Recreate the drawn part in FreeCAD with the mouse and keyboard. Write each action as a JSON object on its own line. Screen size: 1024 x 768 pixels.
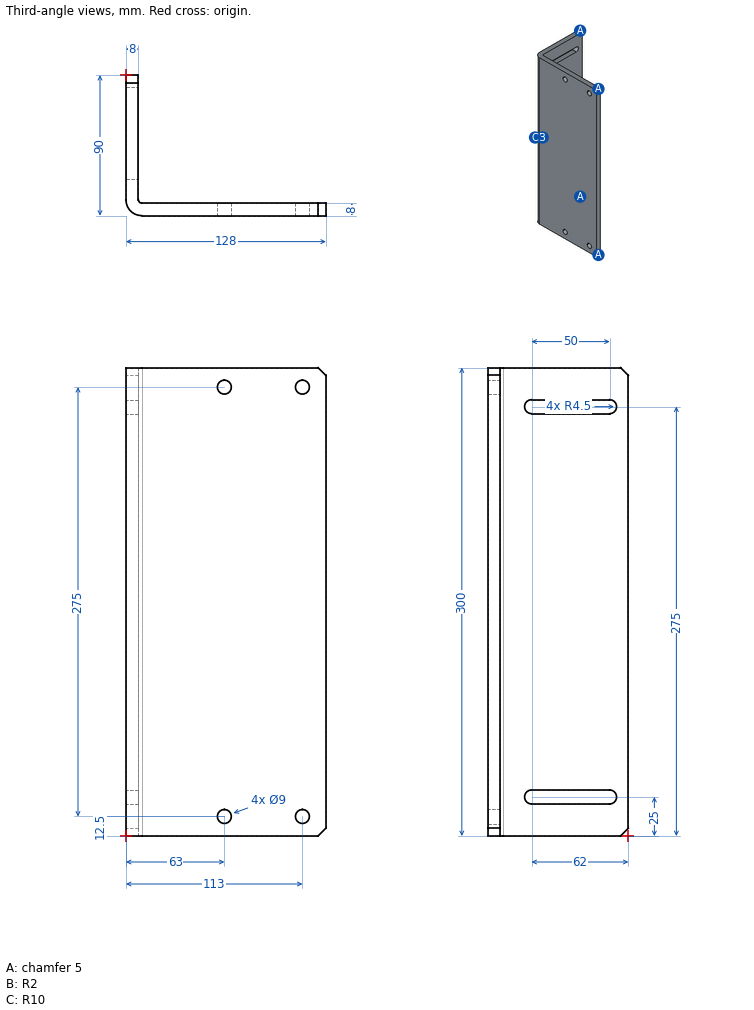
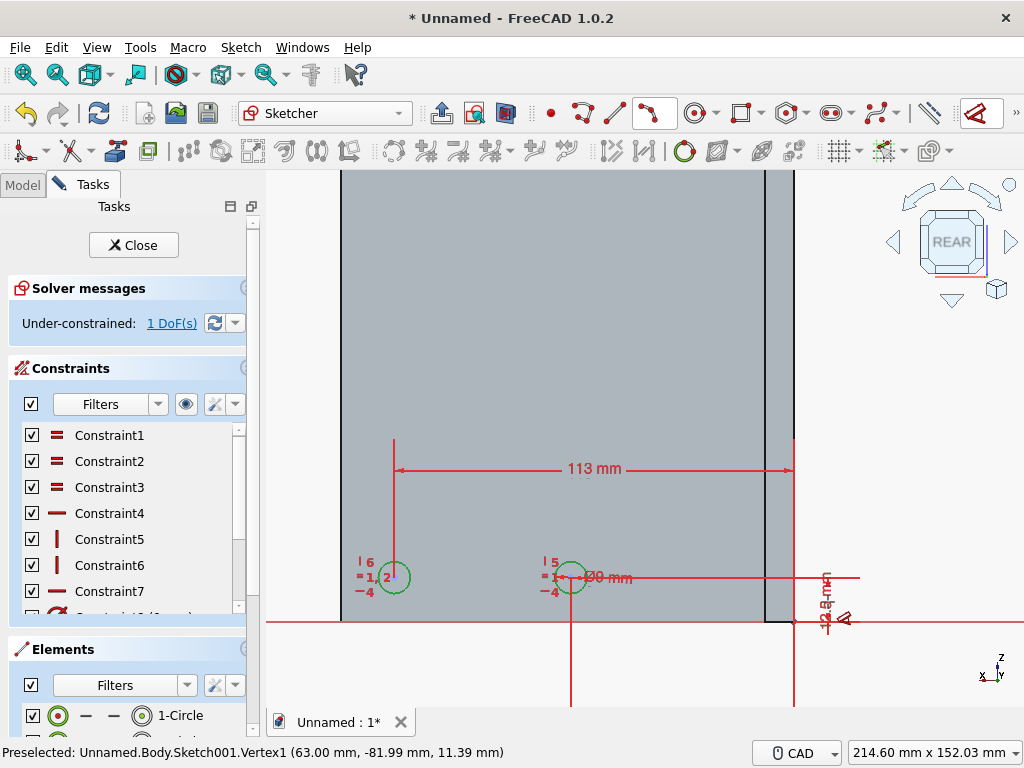
{"action": "left_click", "coordinate": [571, 578]}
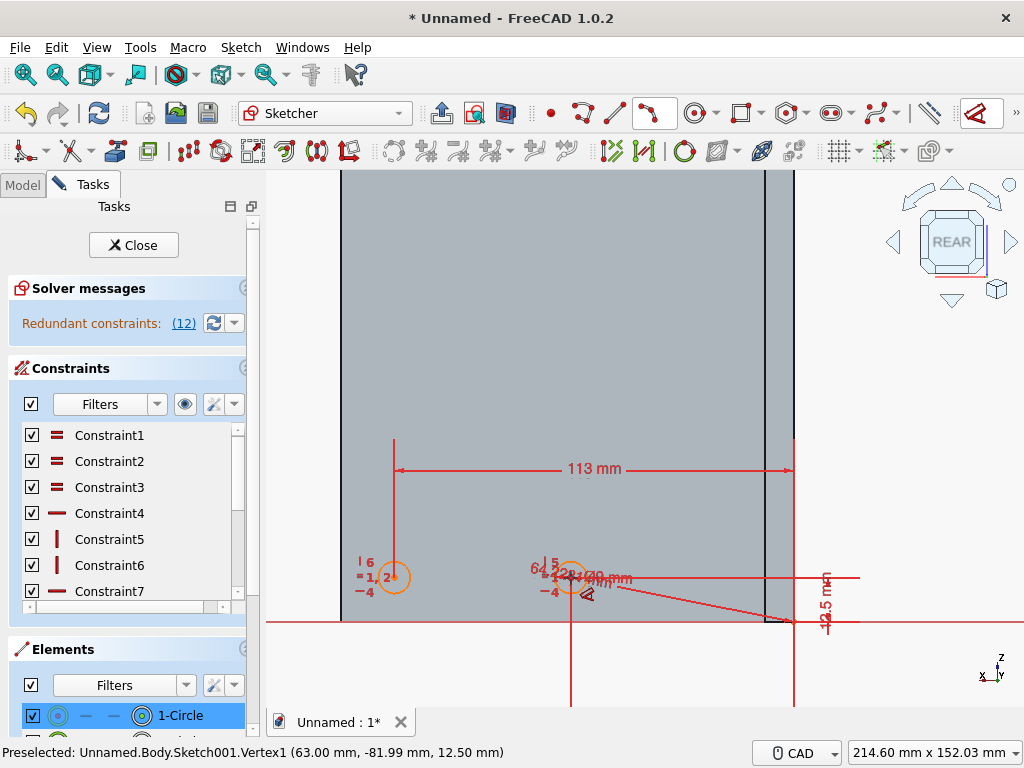
{"action": "scroll", "coordinate": [572, 582], "scroll_direction": "down", "scroll_amount": 6}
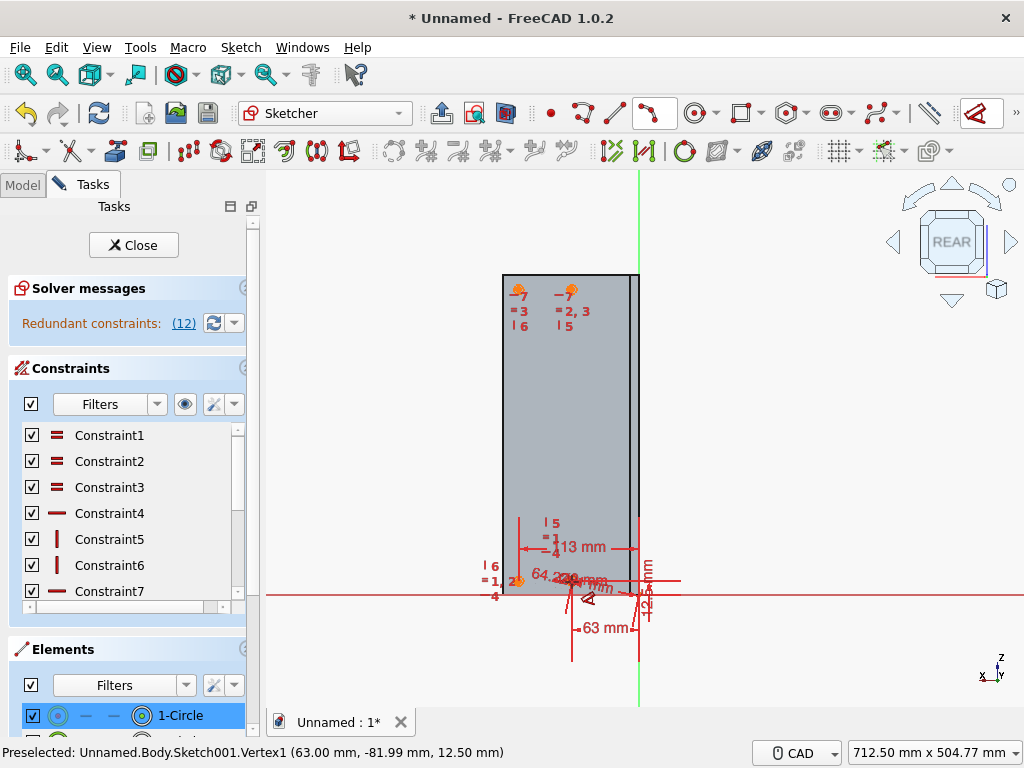
{"action": "left_click", "coordinate": [572, 290]}
{"action": "left_click", "coordinate": [538, 435]}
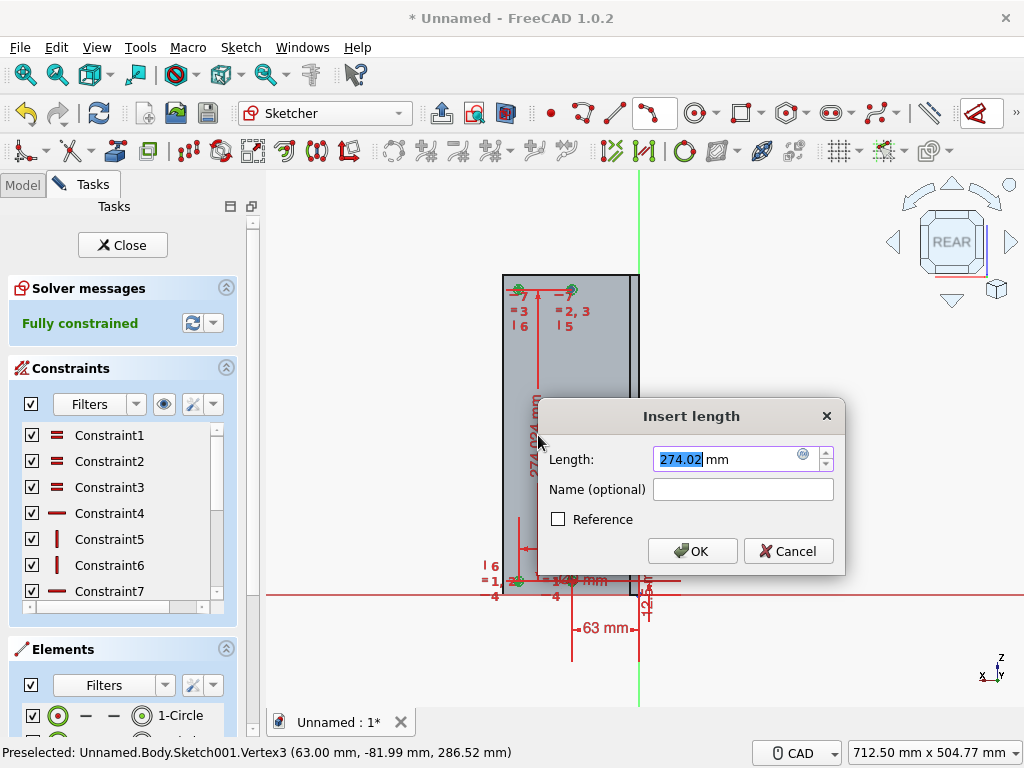
{"action": "type", "text": "275"}
{"action": "key", "text": "Return"}
{"action": "key", "text": "Escape"}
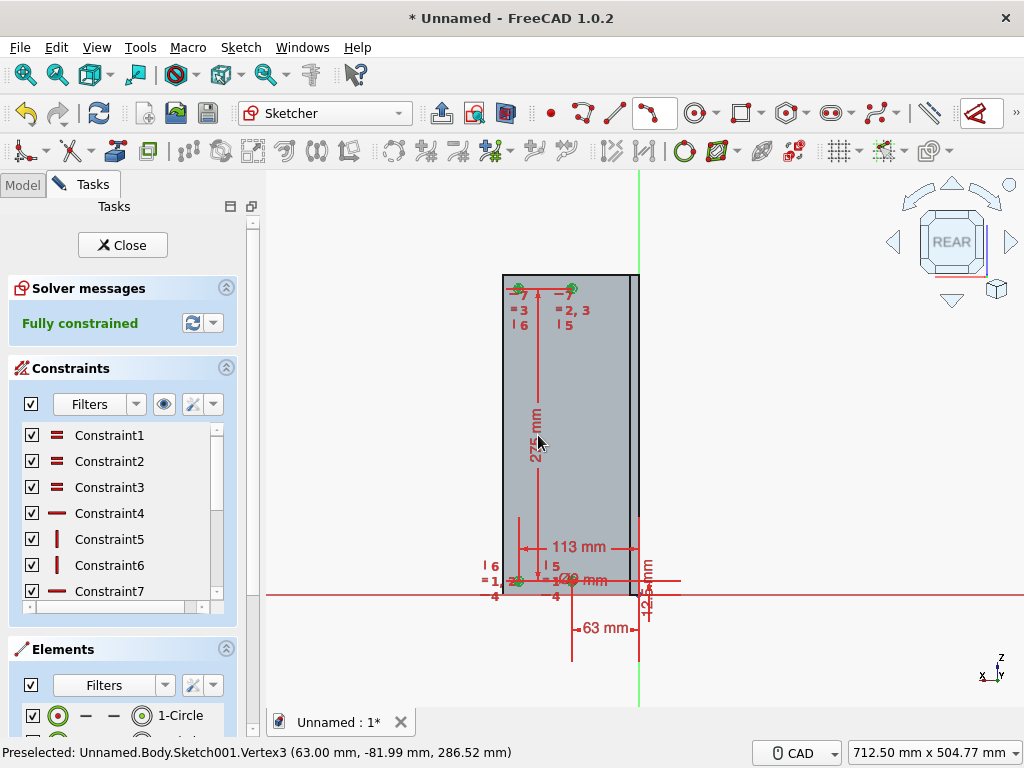
{"action": "left_click", "coordinate": [123, 245]}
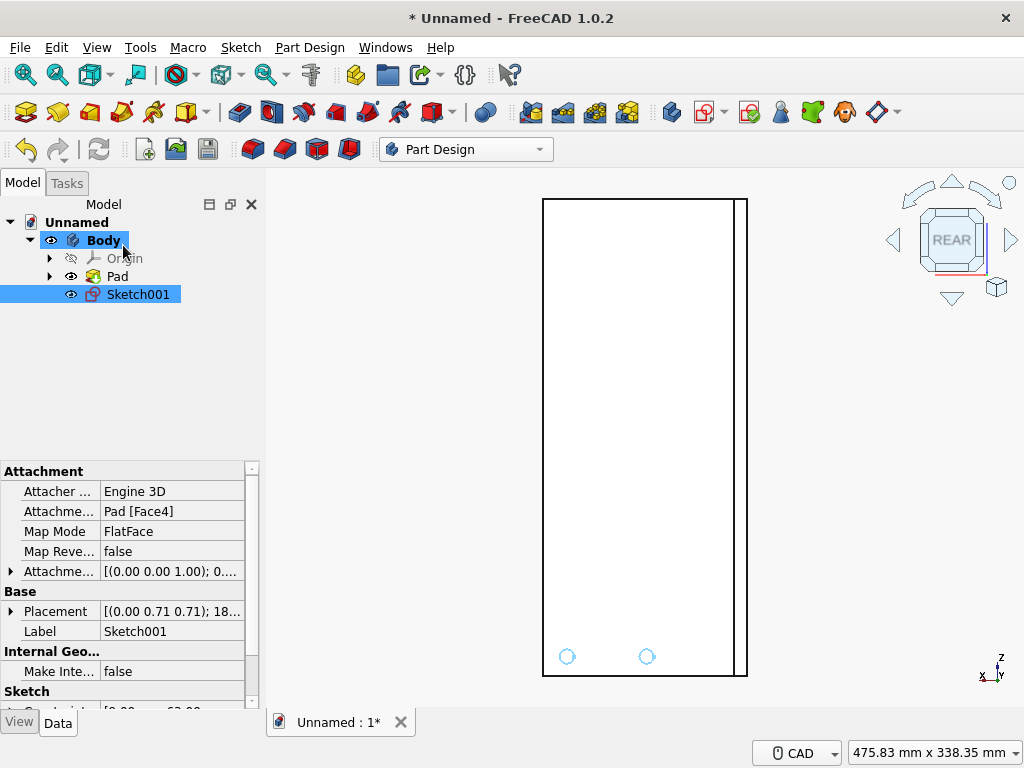
{"action": "left_click", "coordinate": [240, 112]}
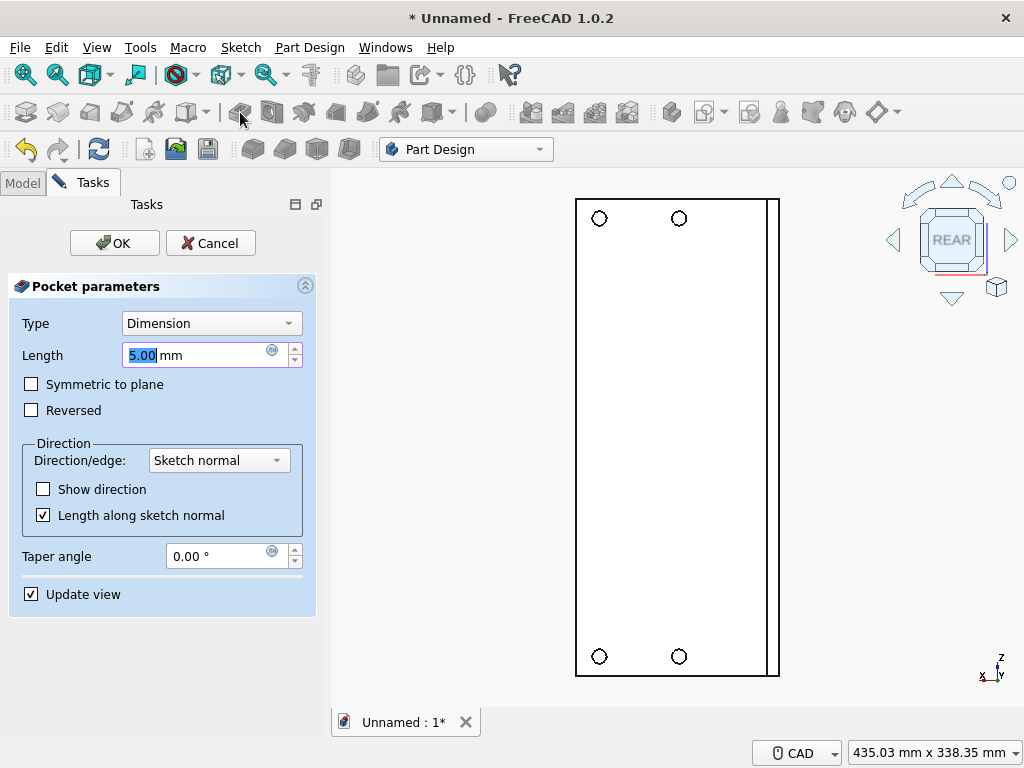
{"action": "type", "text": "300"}
{"action": "key", "text": "Tab"}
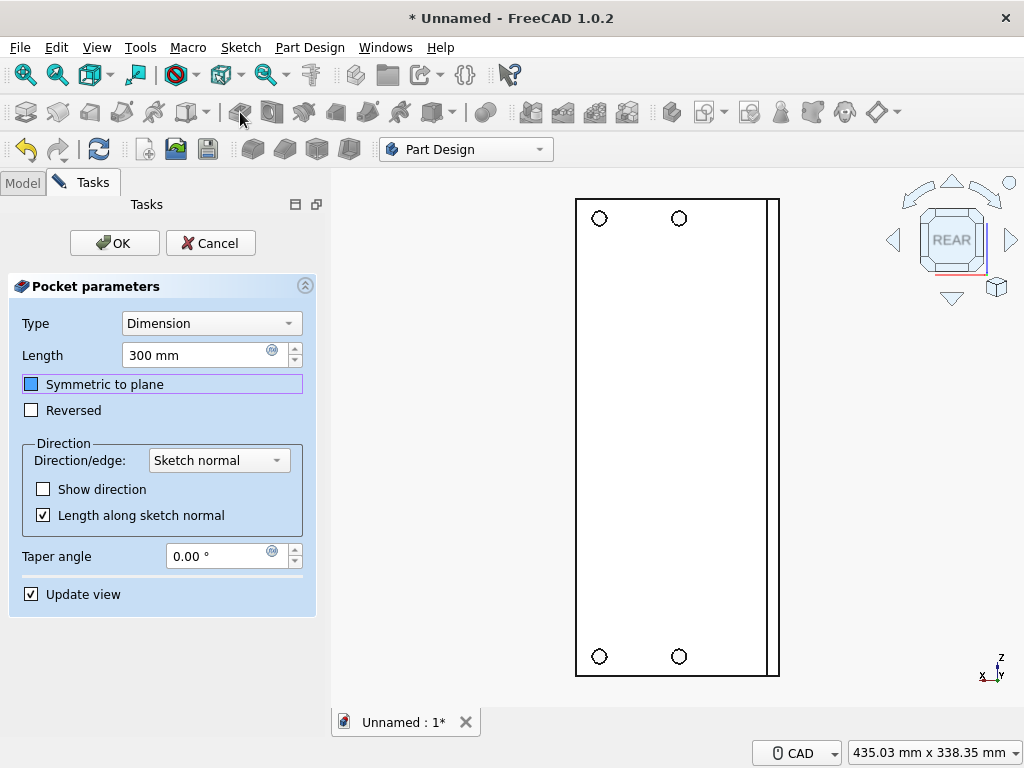
{"action": "left_click", "coordinate": [115, 243]}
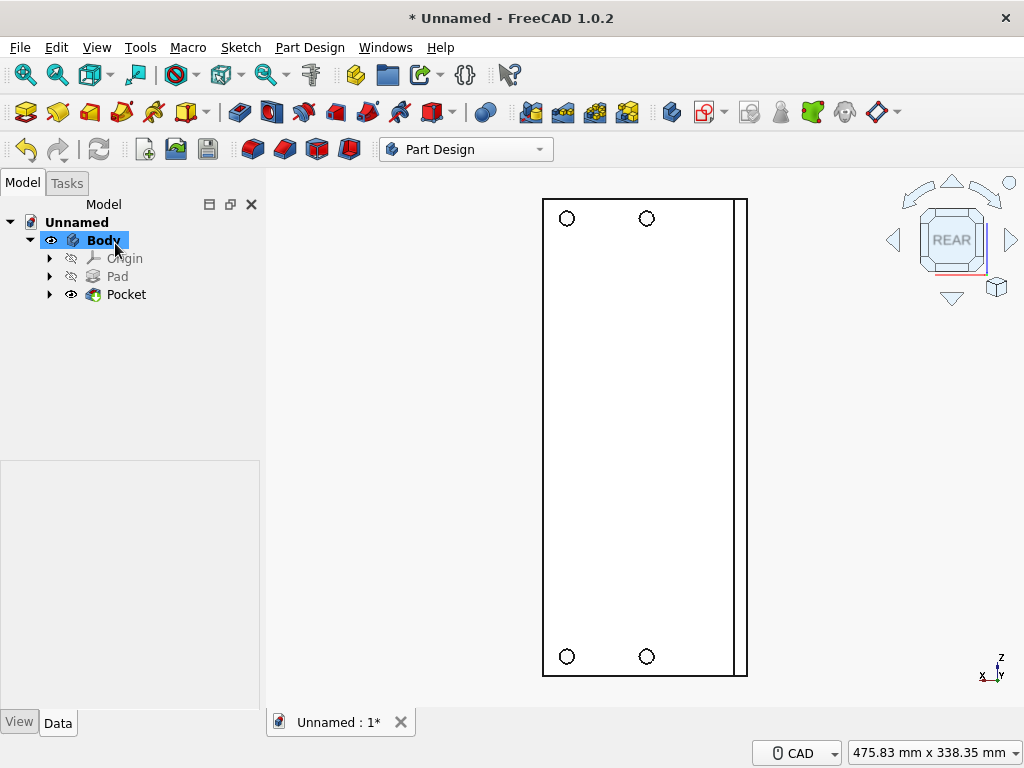
{"action": "key", "text": "0"}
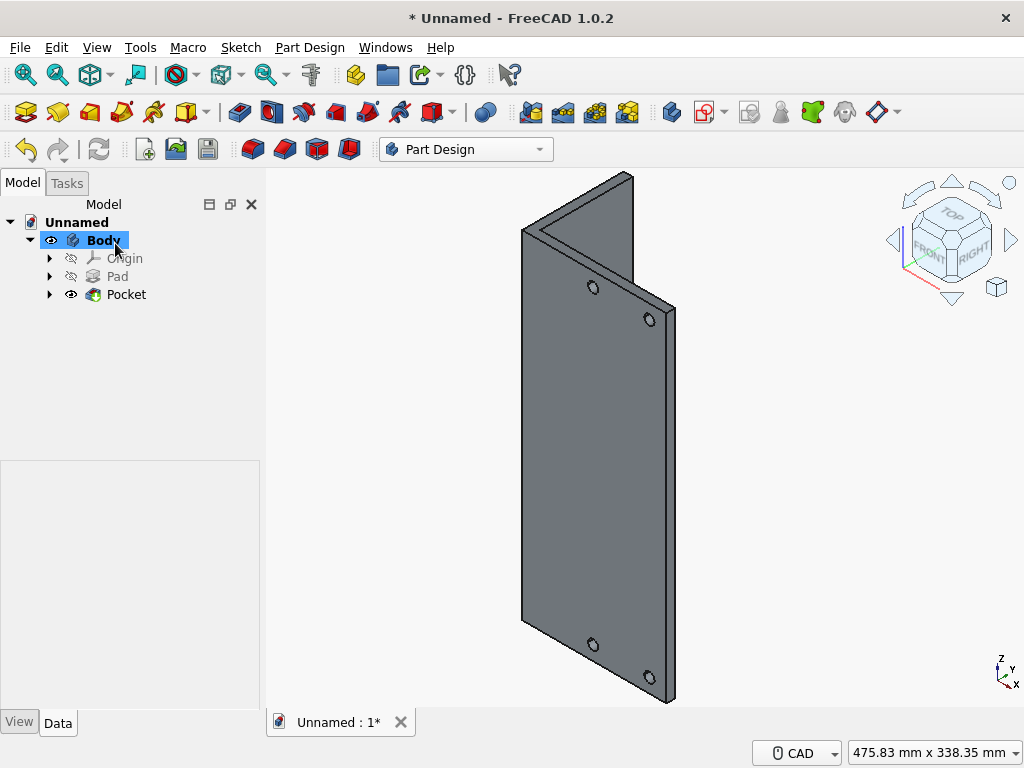
{"action": "key", "text": "3"}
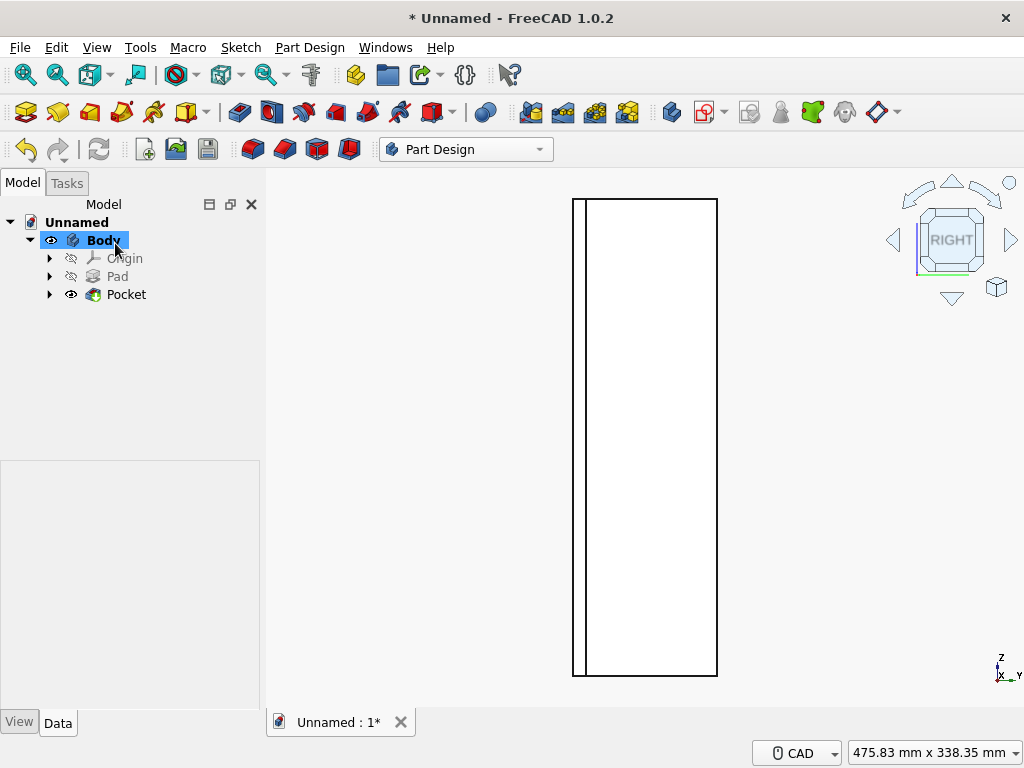
{"action": "left_click", "coordinate": [651, 300]}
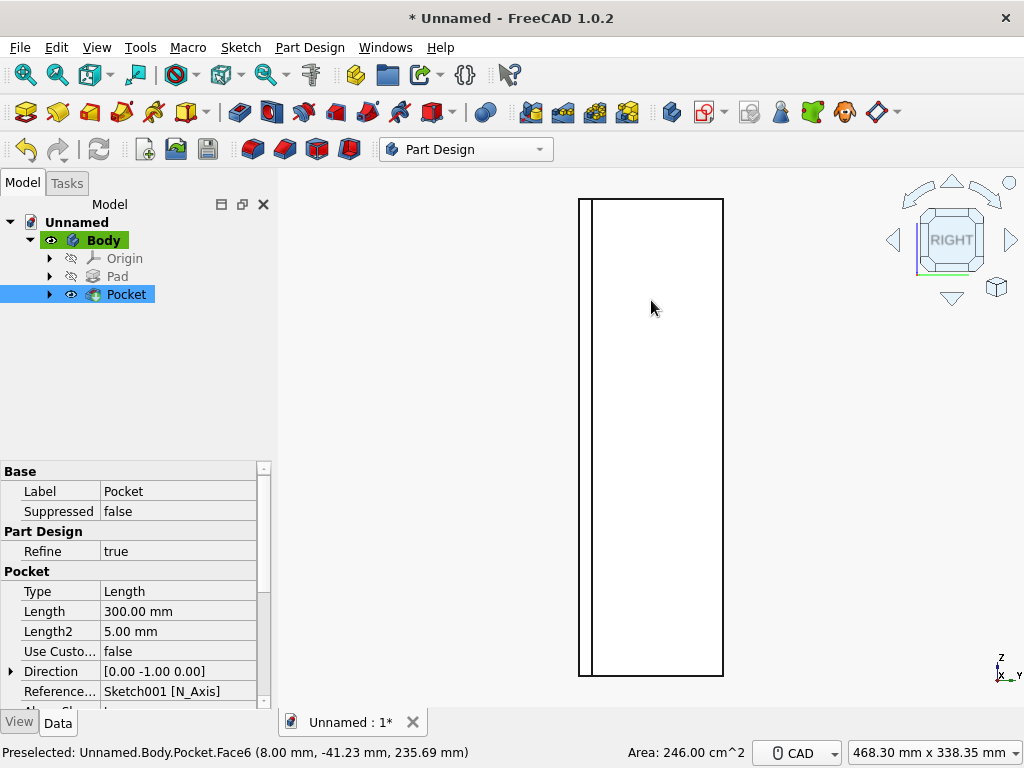
{"action": "left_click", "coordinate": [704, 112]}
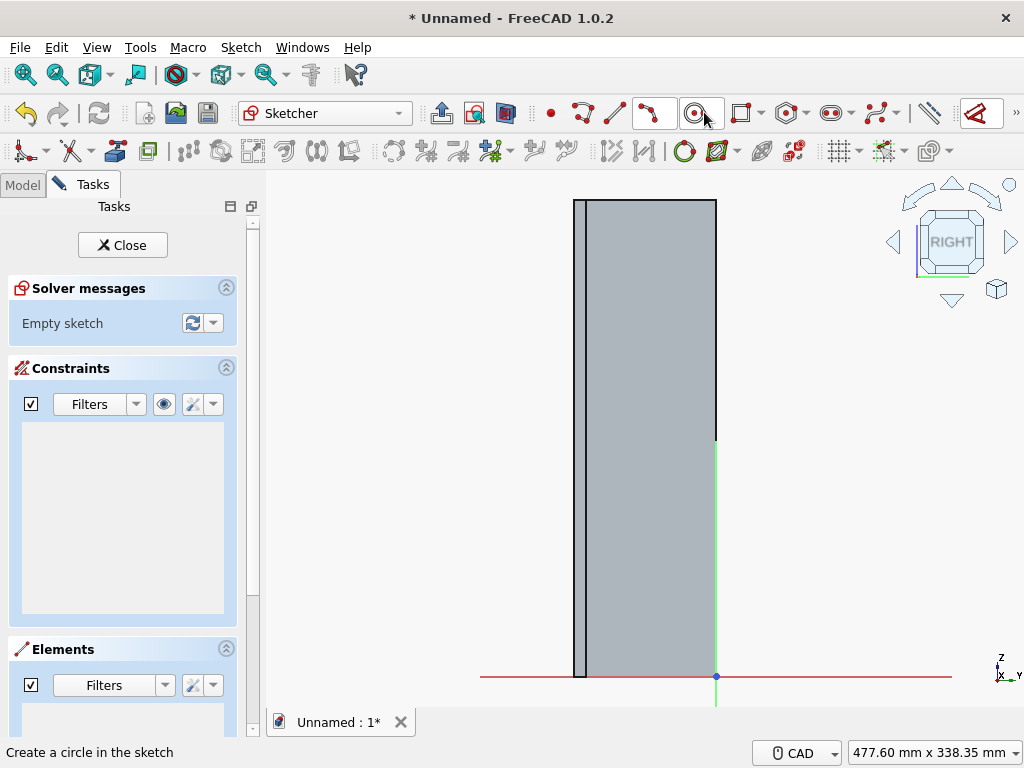
{"action": "key", "text": "q s"}